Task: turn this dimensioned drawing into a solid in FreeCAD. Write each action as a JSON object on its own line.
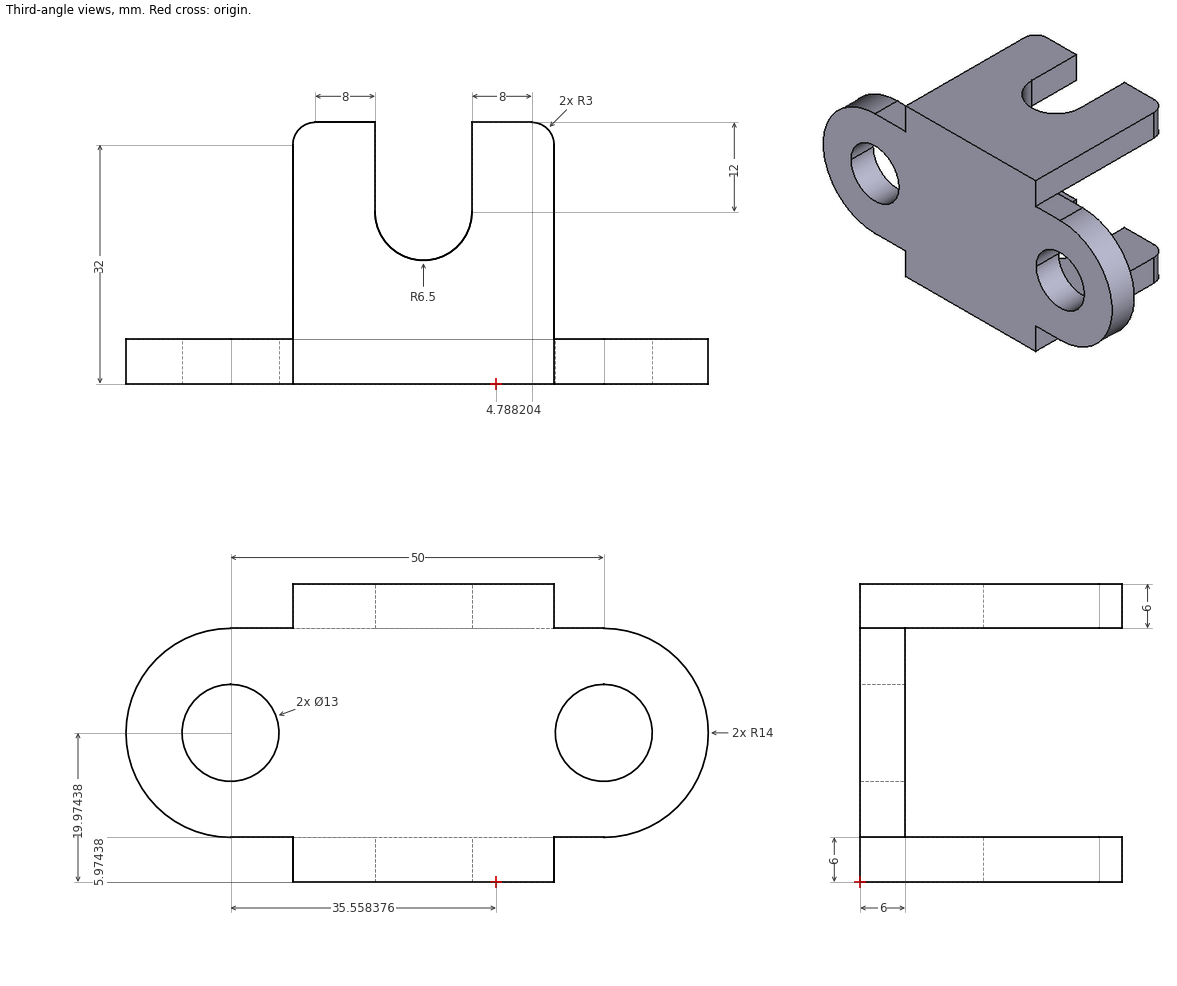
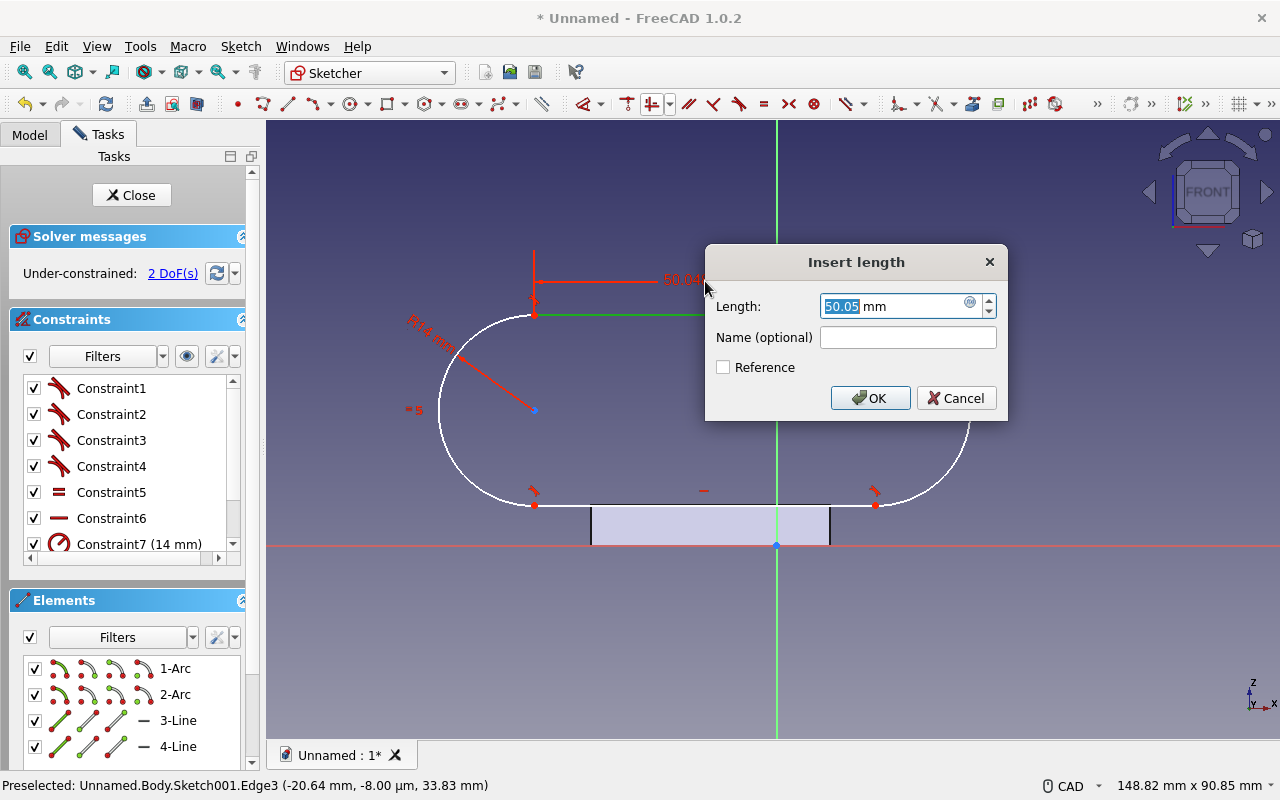
{"action": "type", "text": "50"}
{"action": "key", "text": "Return"}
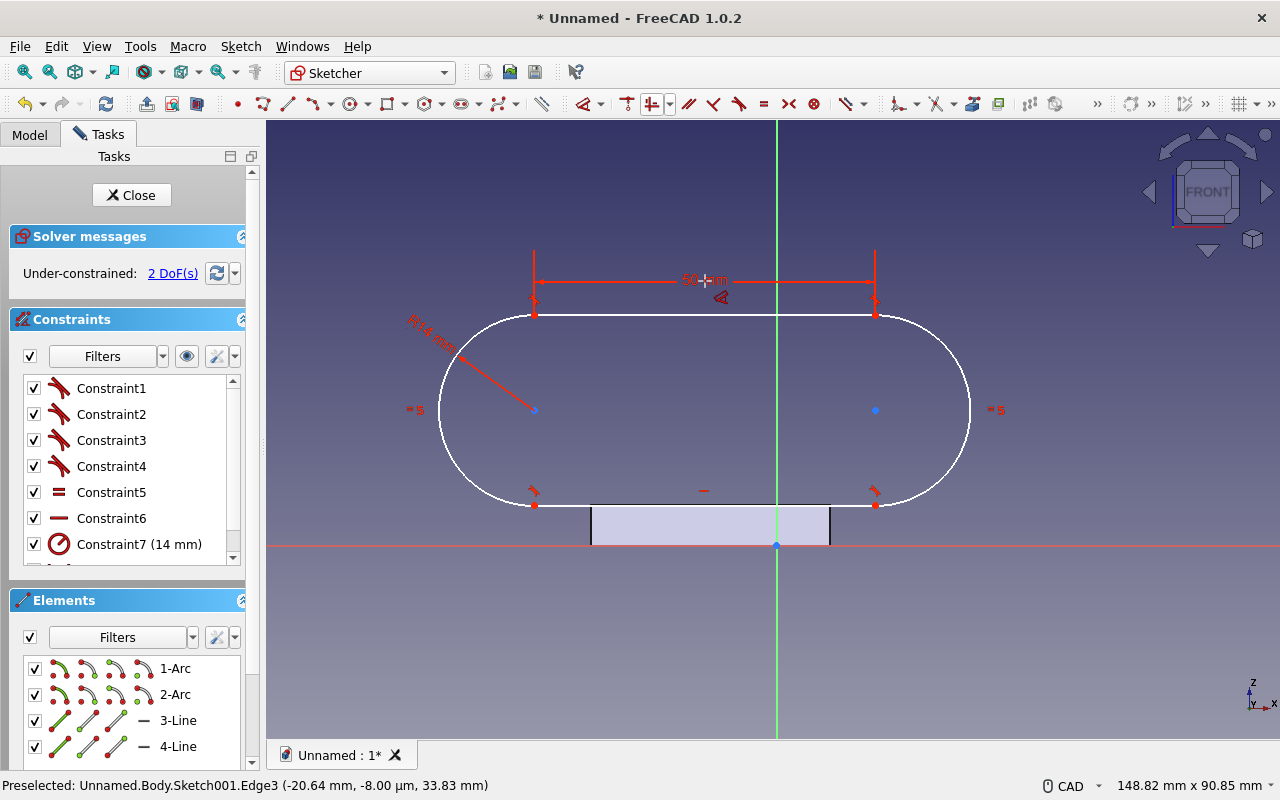
{"action": "left_click", "coordinate": [534, 506]}
{"action": "left_click", "coordinate": [500, 526]}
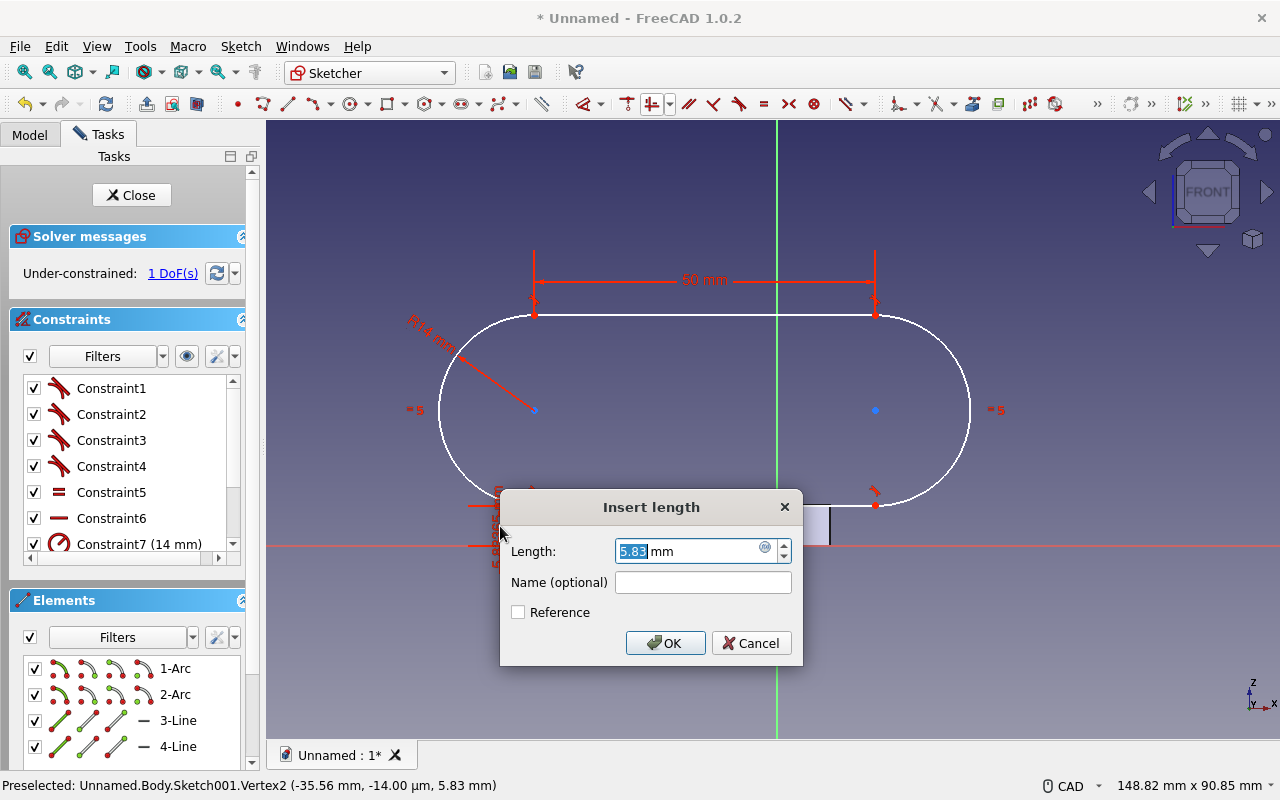
{"action": "type", "text": "5.97438"}
{"action": "key", "text": "Return"}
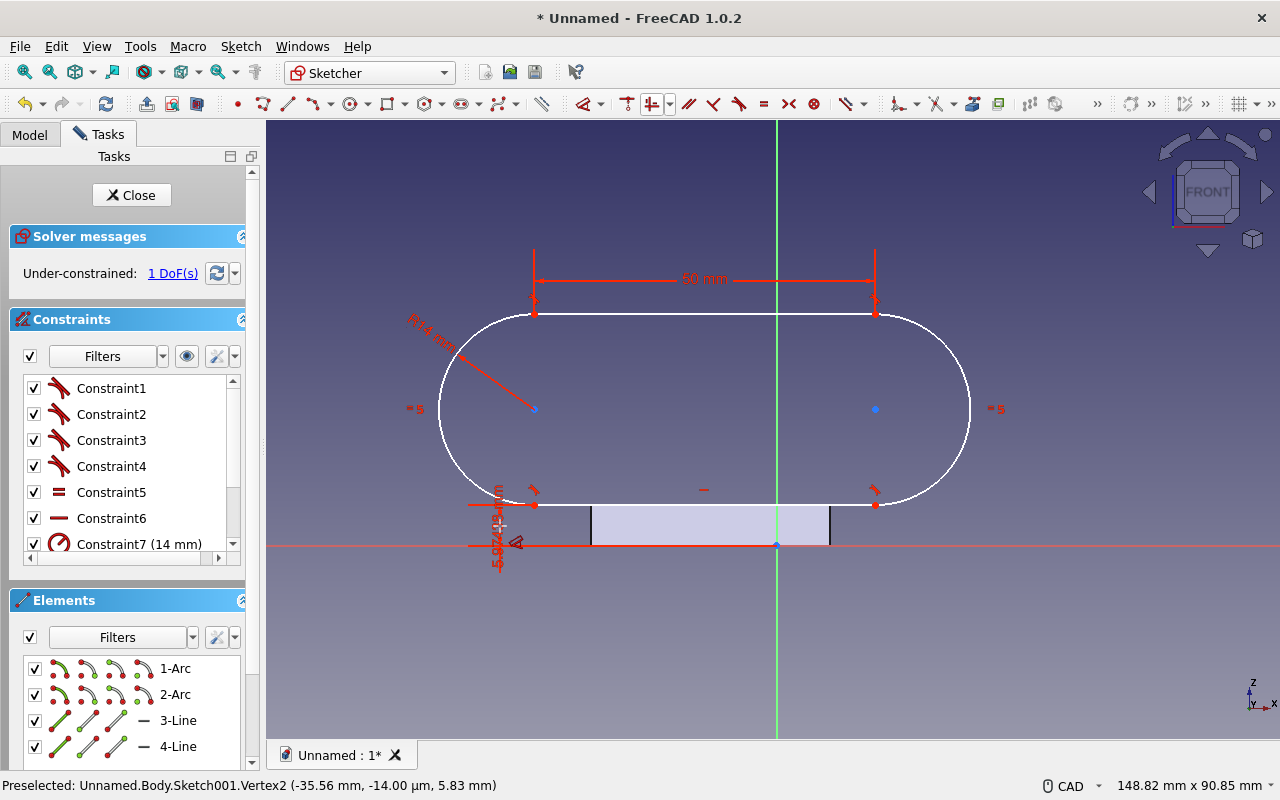
{"action": "left_click", "coordinate": [534, 314]}
{"action": "left_click", "coordinate": [655, 580]}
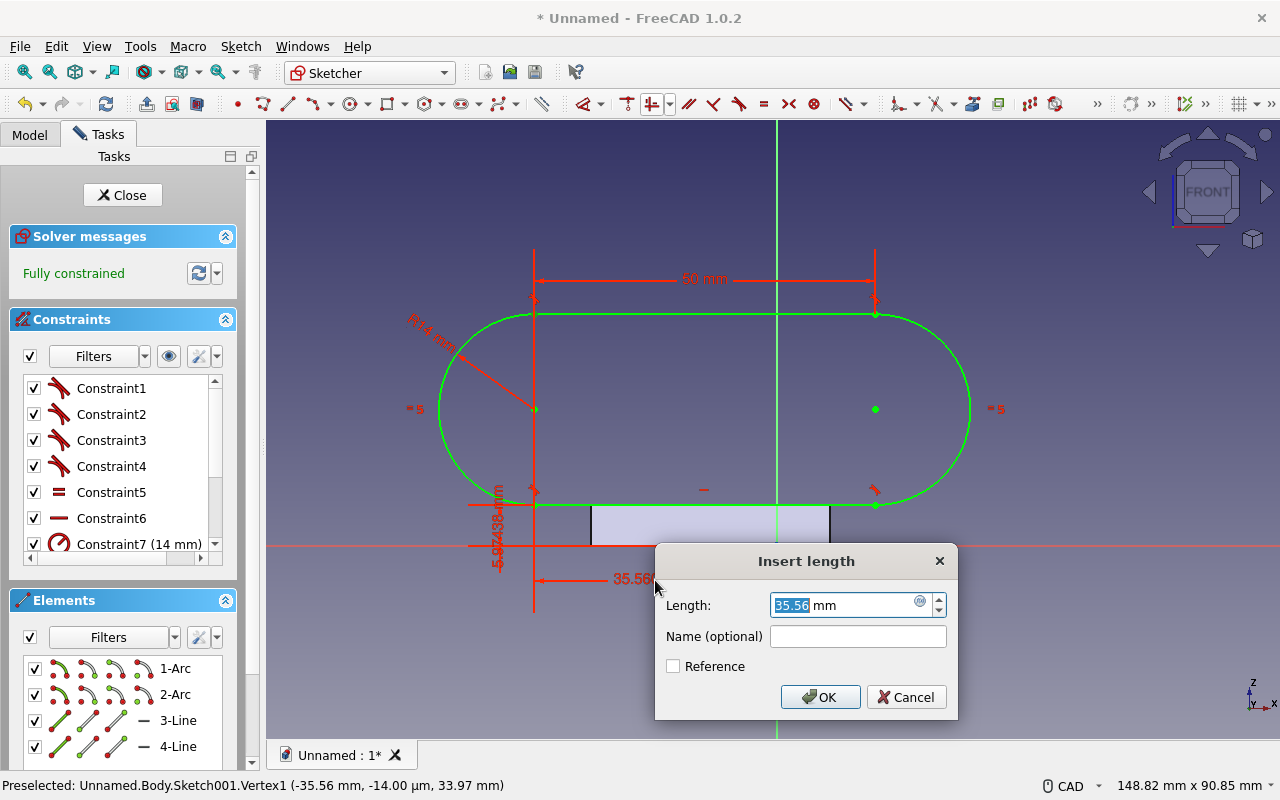
{"action": "type", "text": "35.558376"}
{"action": "key", "text": "Return"}
{"action": "key", "text": "Escape"}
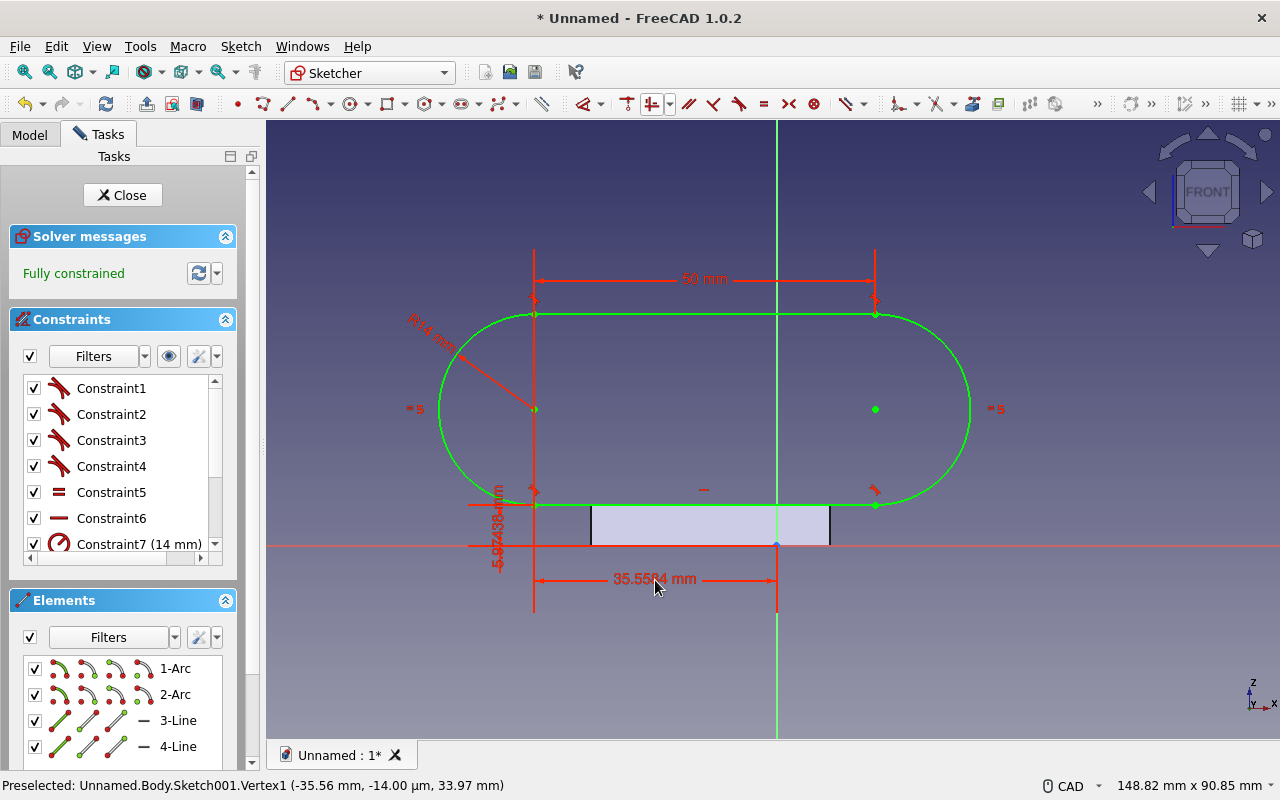
{"action": "left_click", "coordinate": [123, 195]}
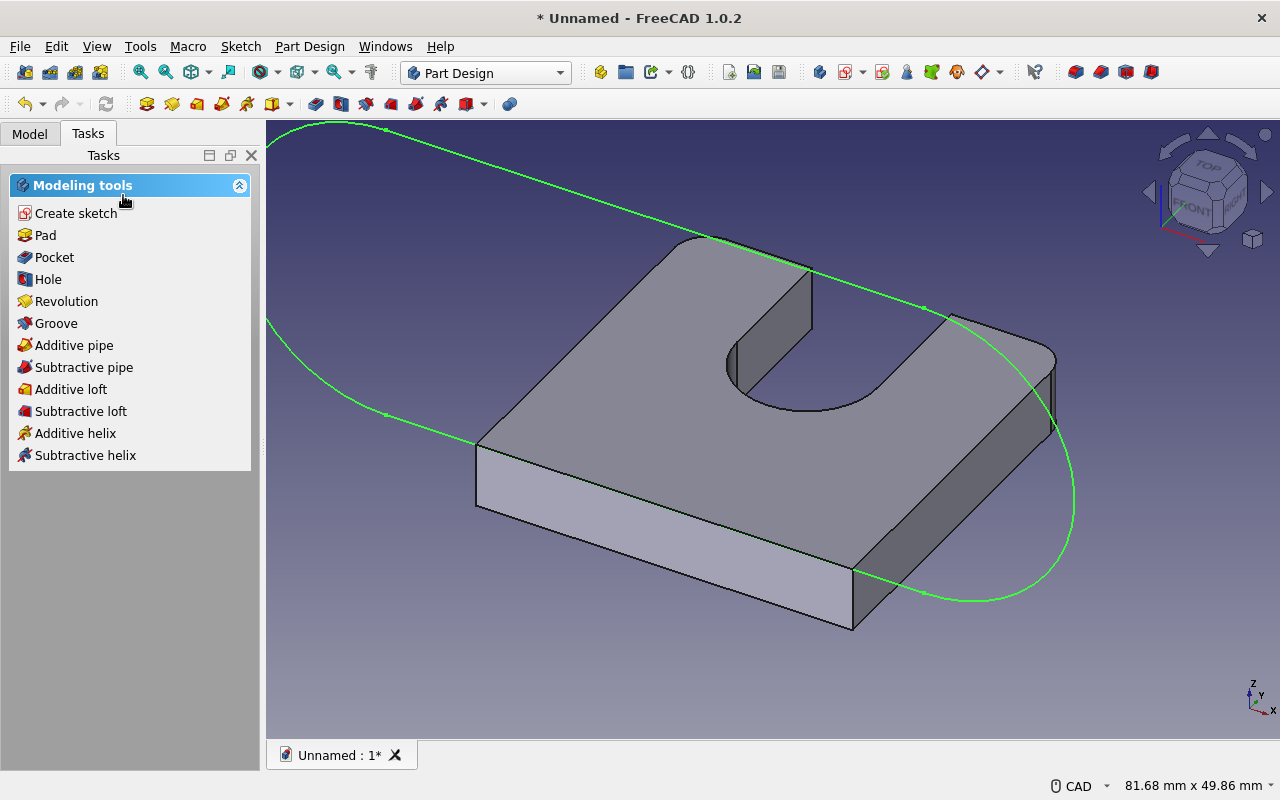
{"action": "left_click", "coordinate": [147, 104]}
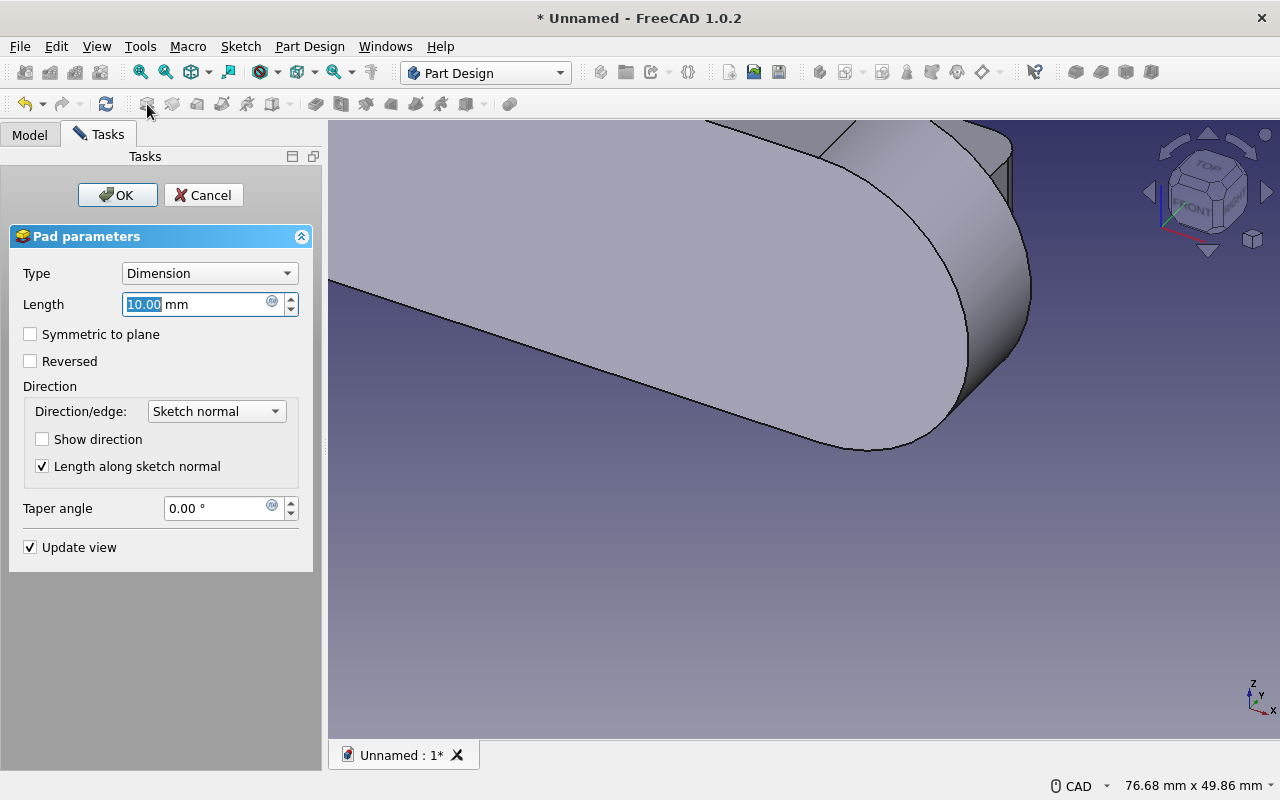
{"action": "type", "text": "6"}
{"action": "key", "text": "Tab"}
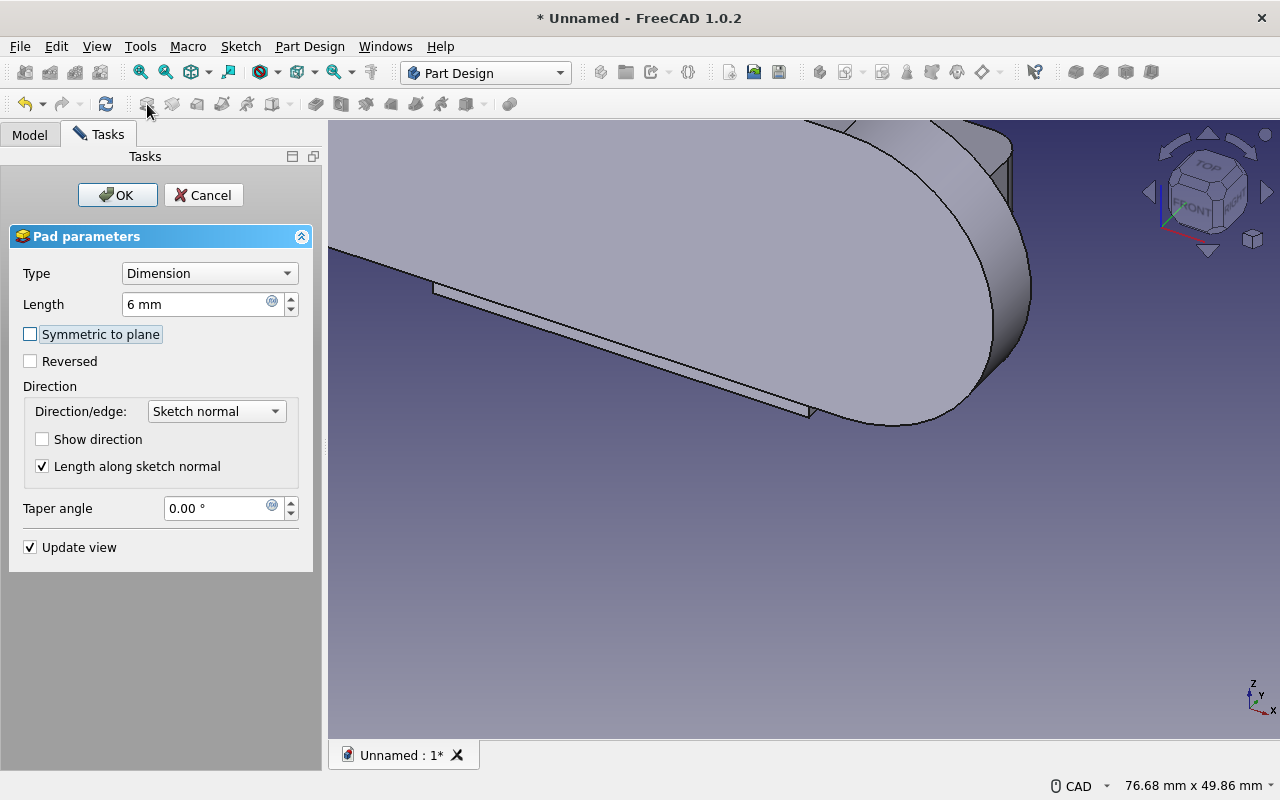
{"action": "left_click", "coordinate": [31, 361]}